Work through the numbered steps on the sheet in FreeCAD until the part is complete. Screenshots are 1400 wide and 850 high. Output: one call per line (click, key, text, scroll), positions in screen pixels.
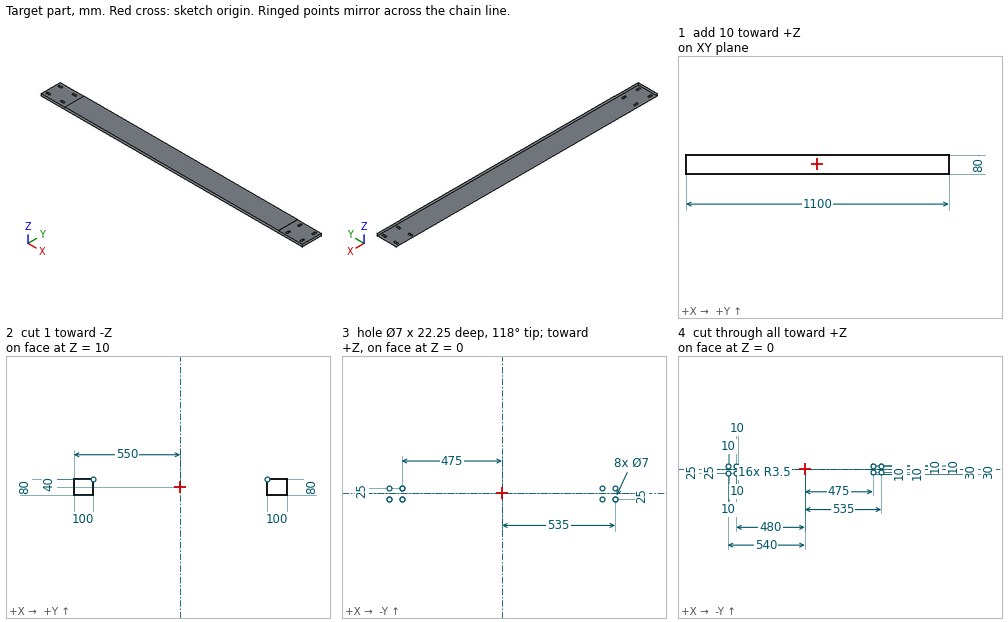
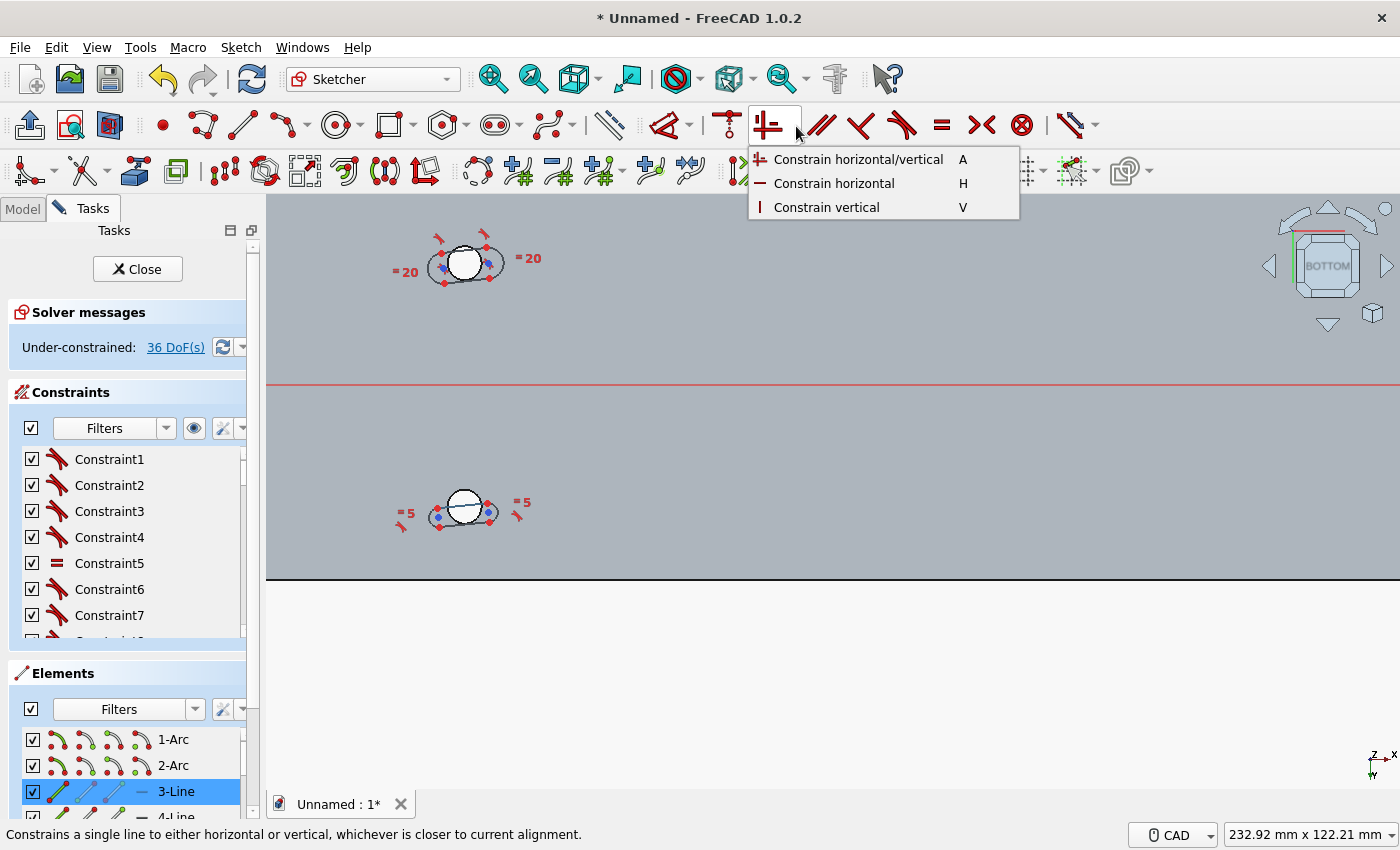
click(884, 183)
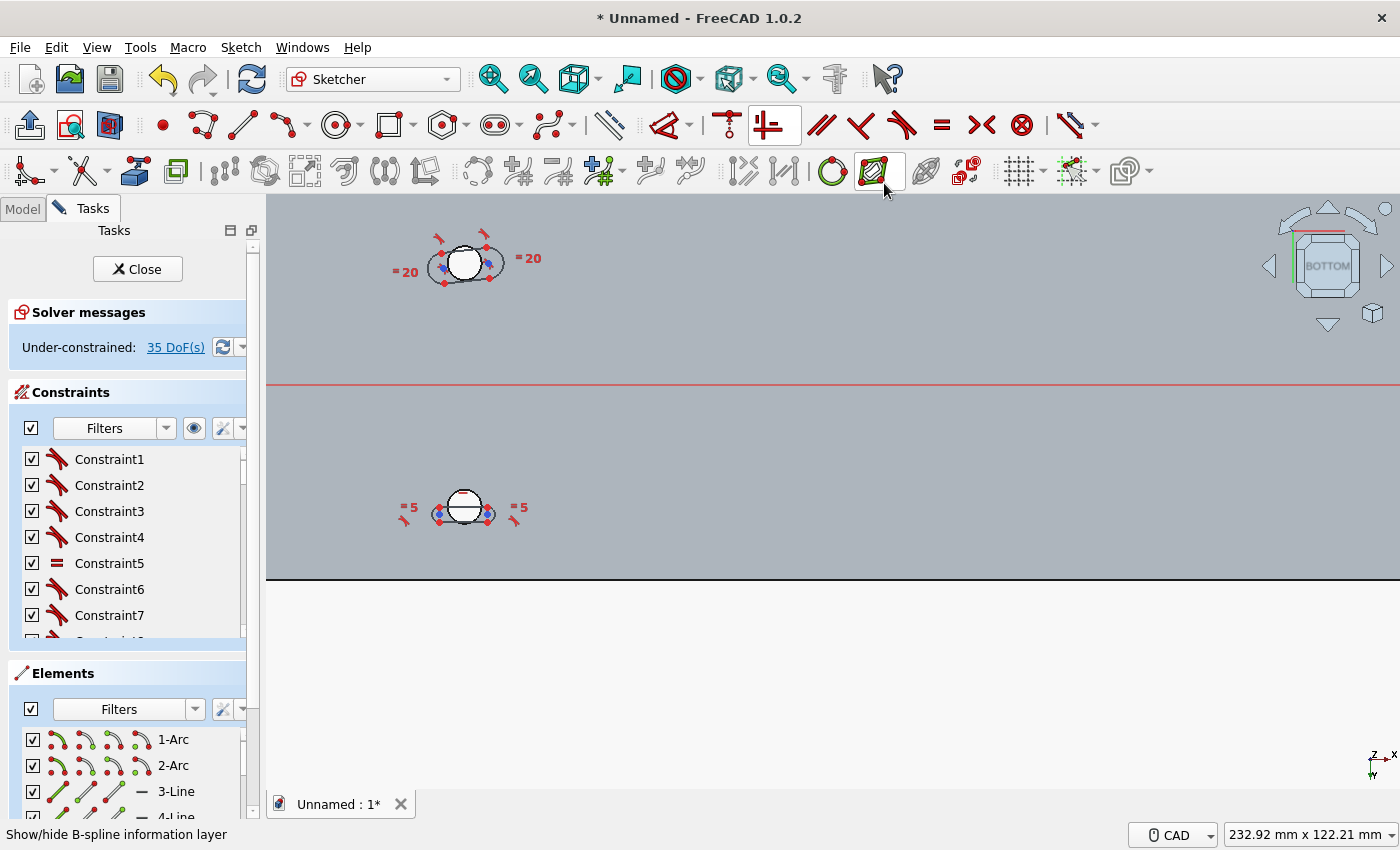
scroll(451, 508, down, 10)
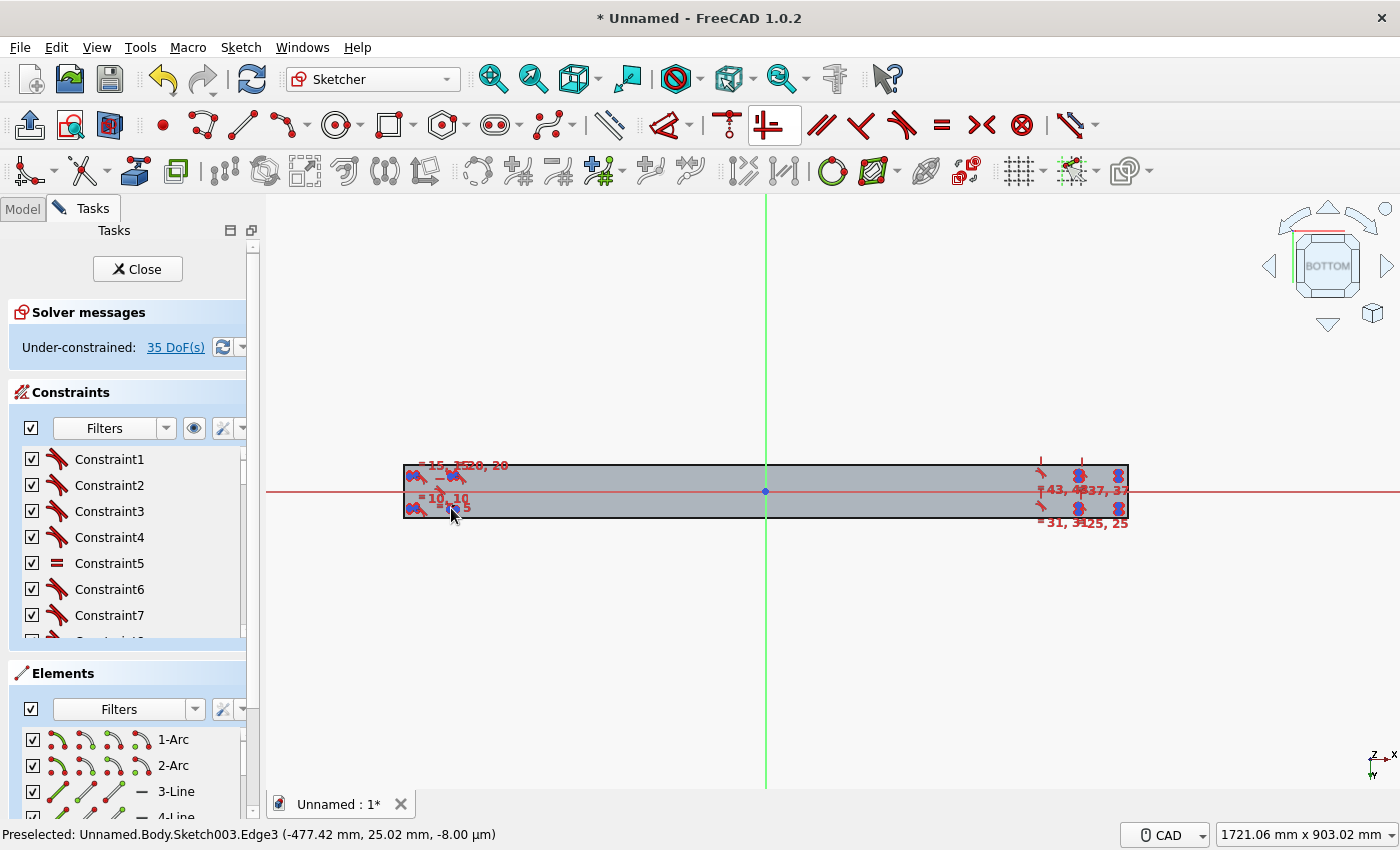
scroll(412, 506, up, 10)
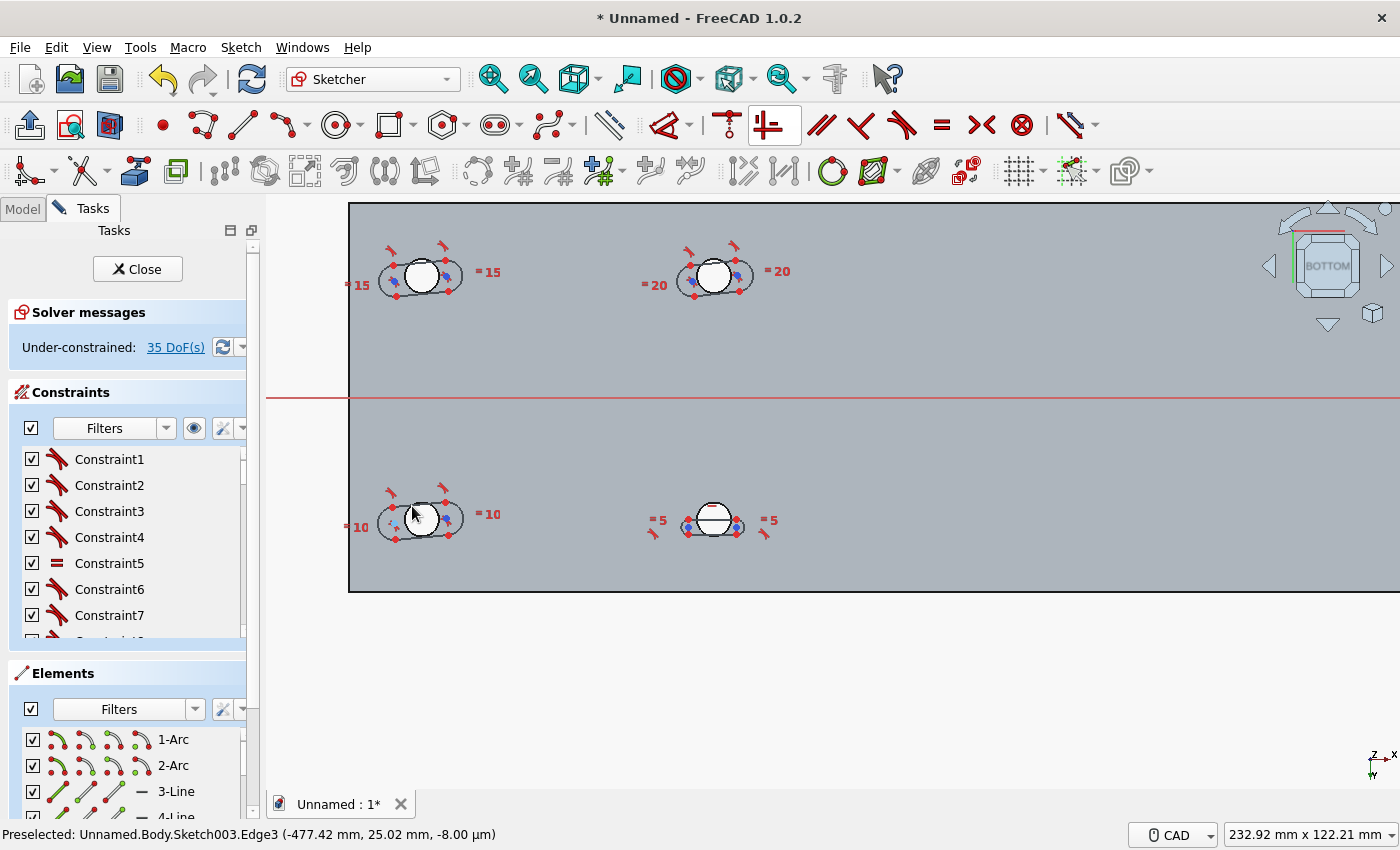
click(409, 506)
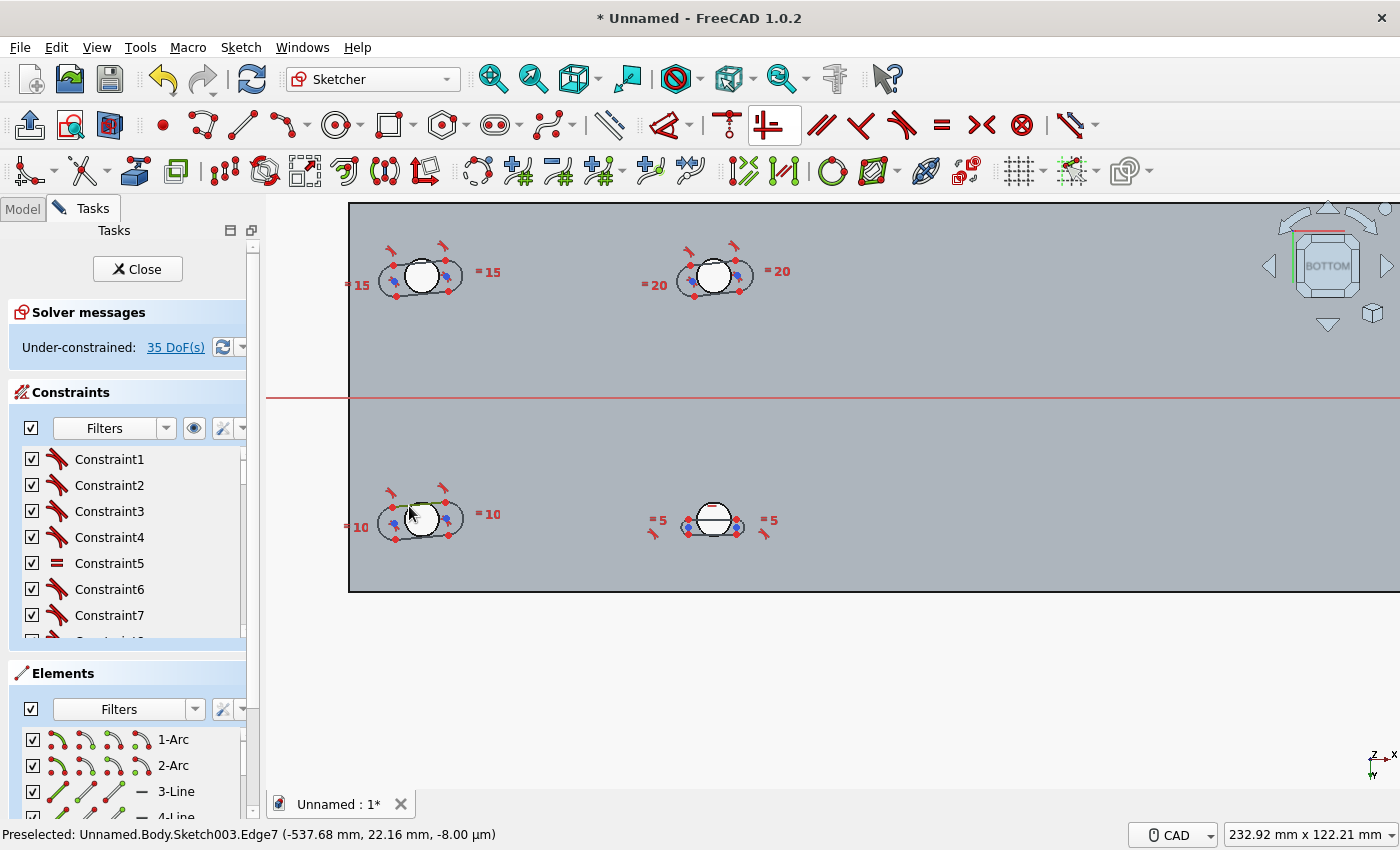
key(h)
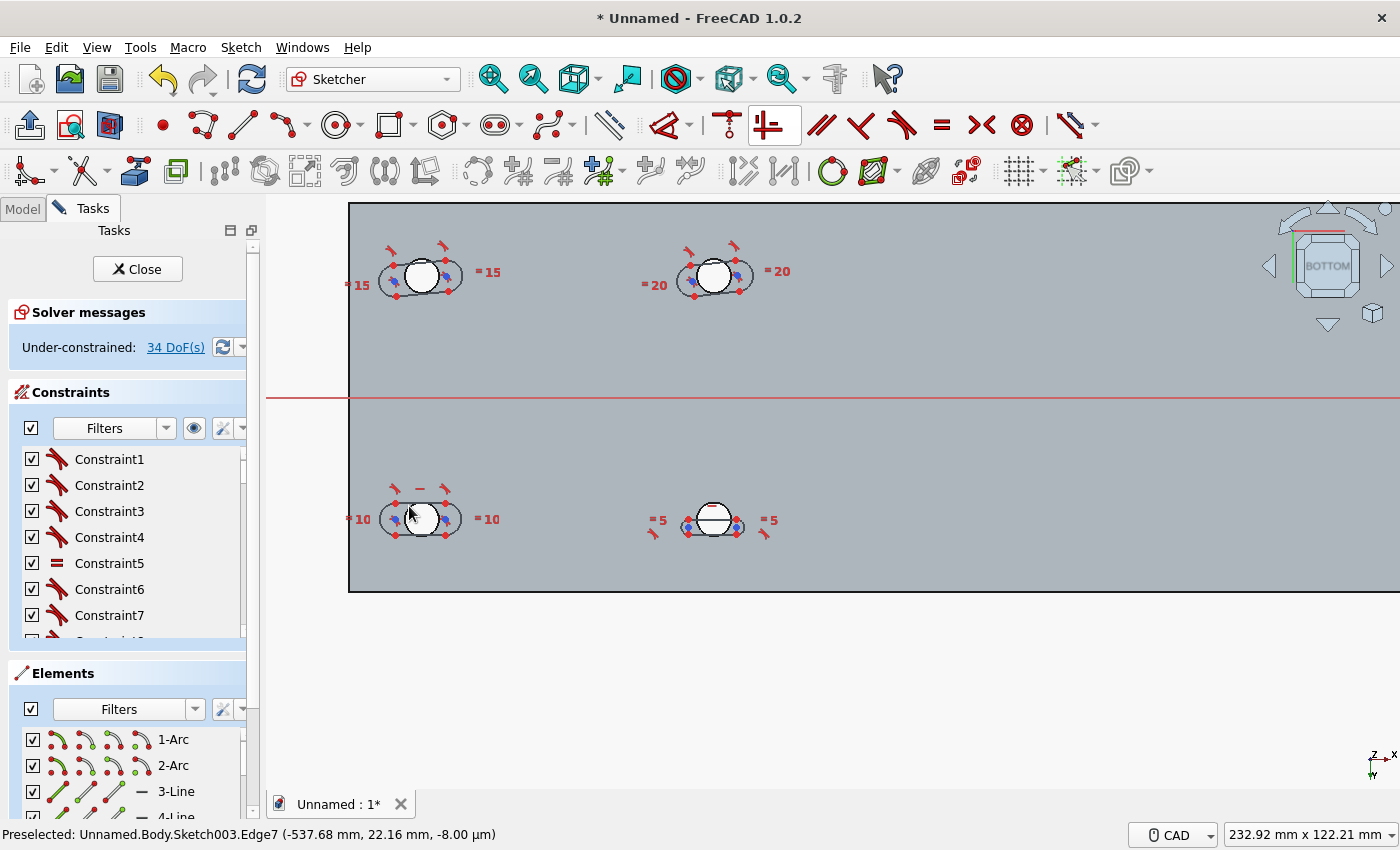
click(409, 264)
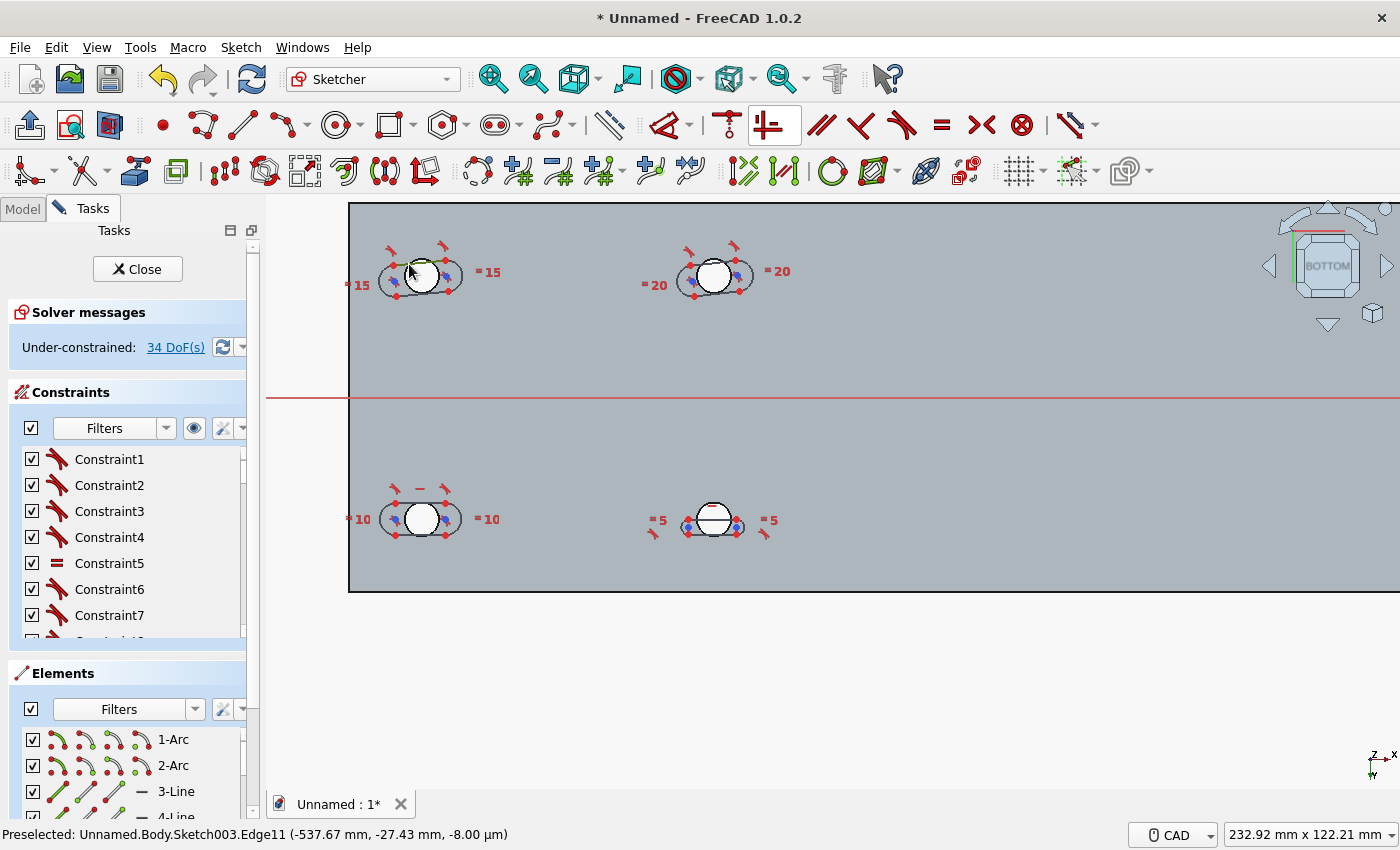
click(796, 126)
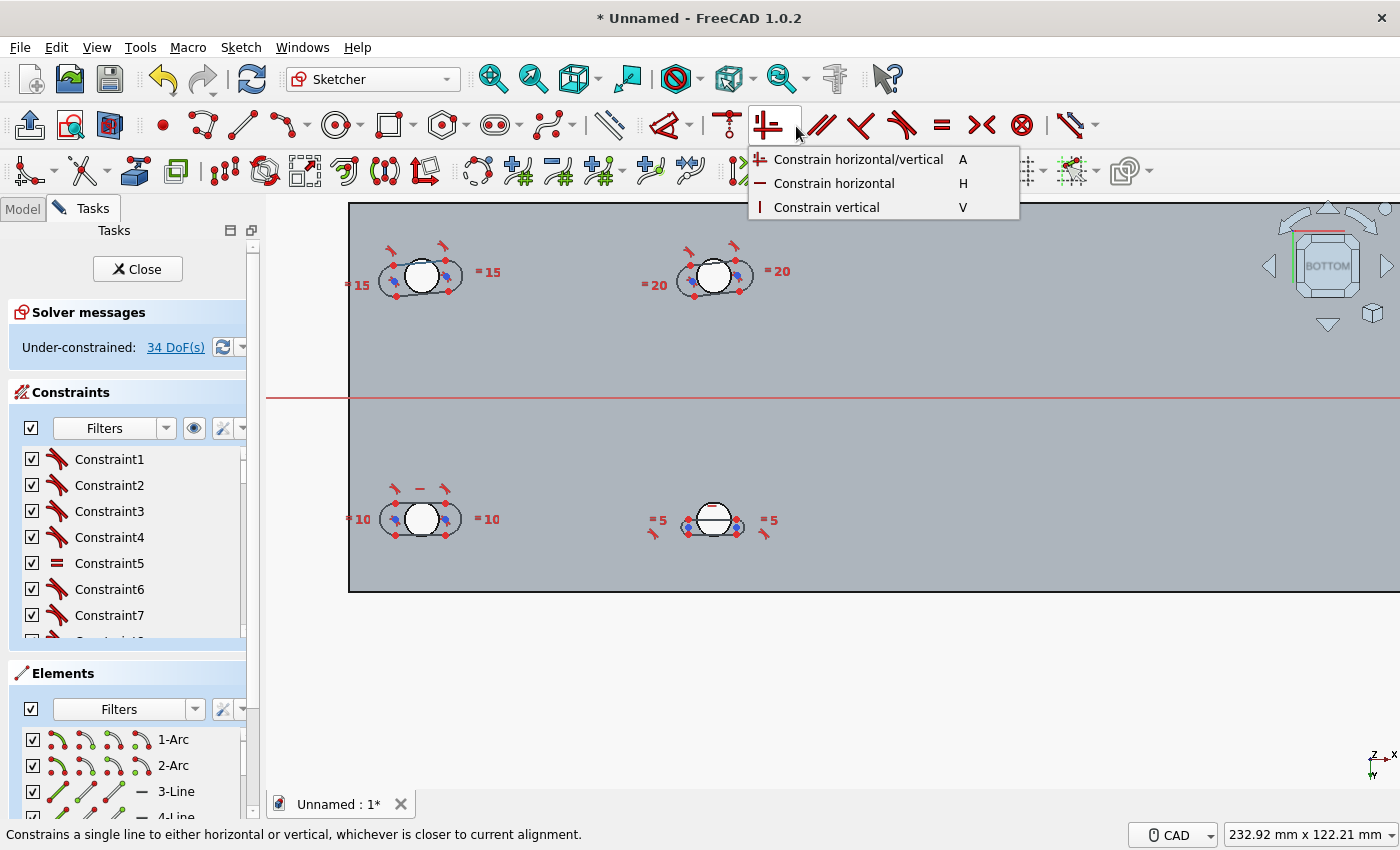
click(884, 183)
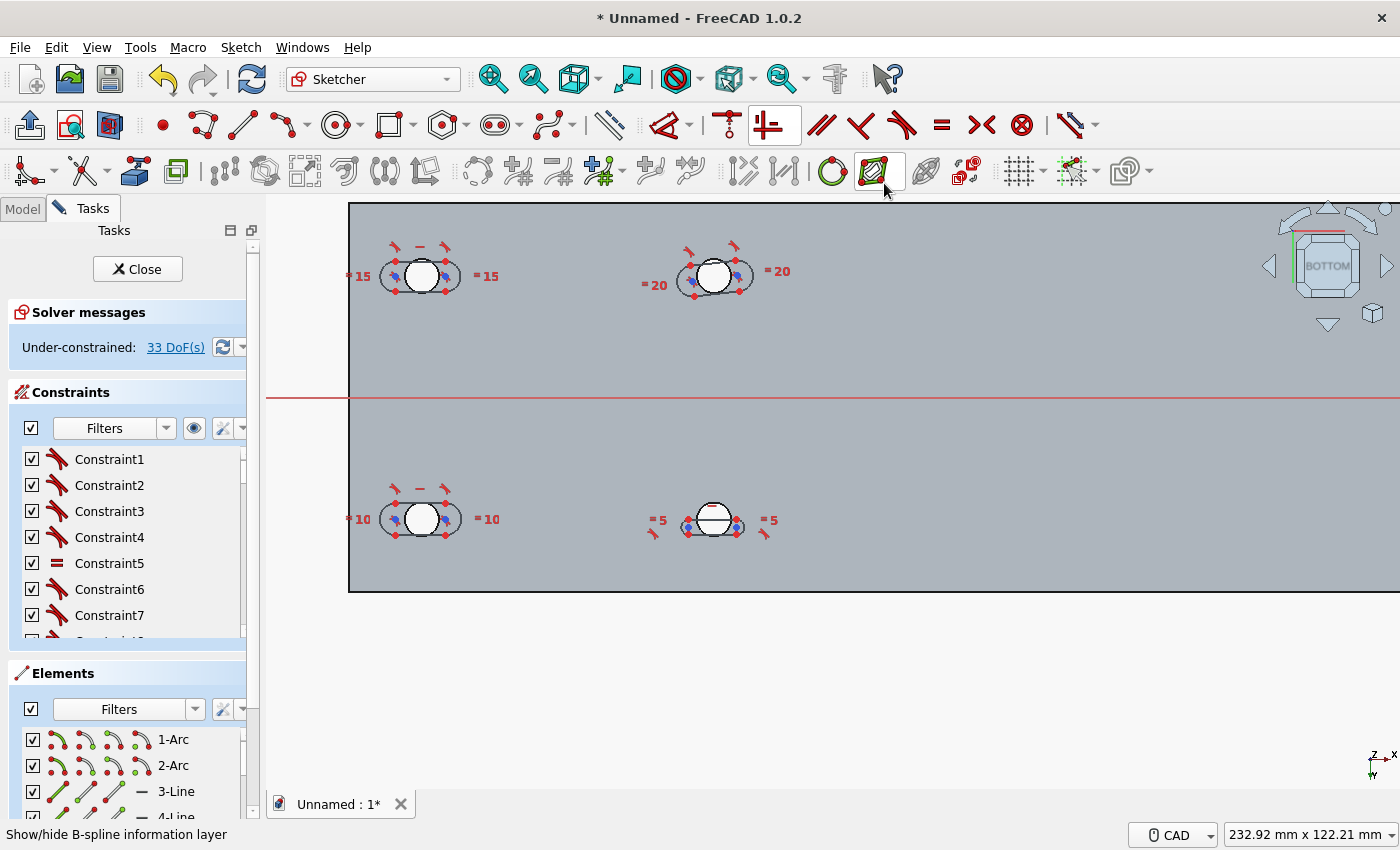
click(704, 264)